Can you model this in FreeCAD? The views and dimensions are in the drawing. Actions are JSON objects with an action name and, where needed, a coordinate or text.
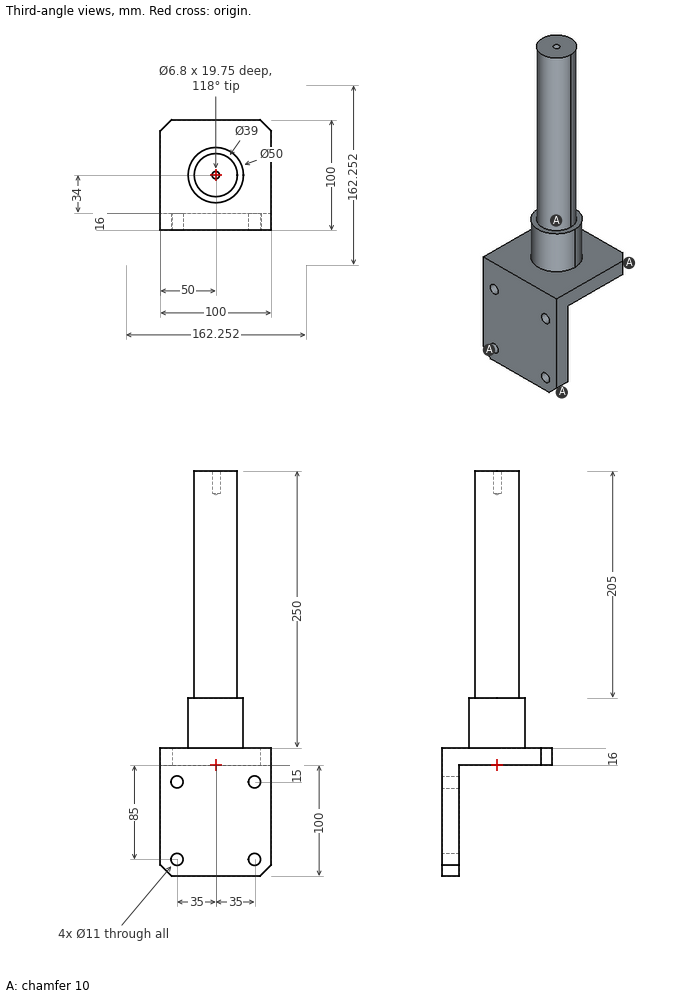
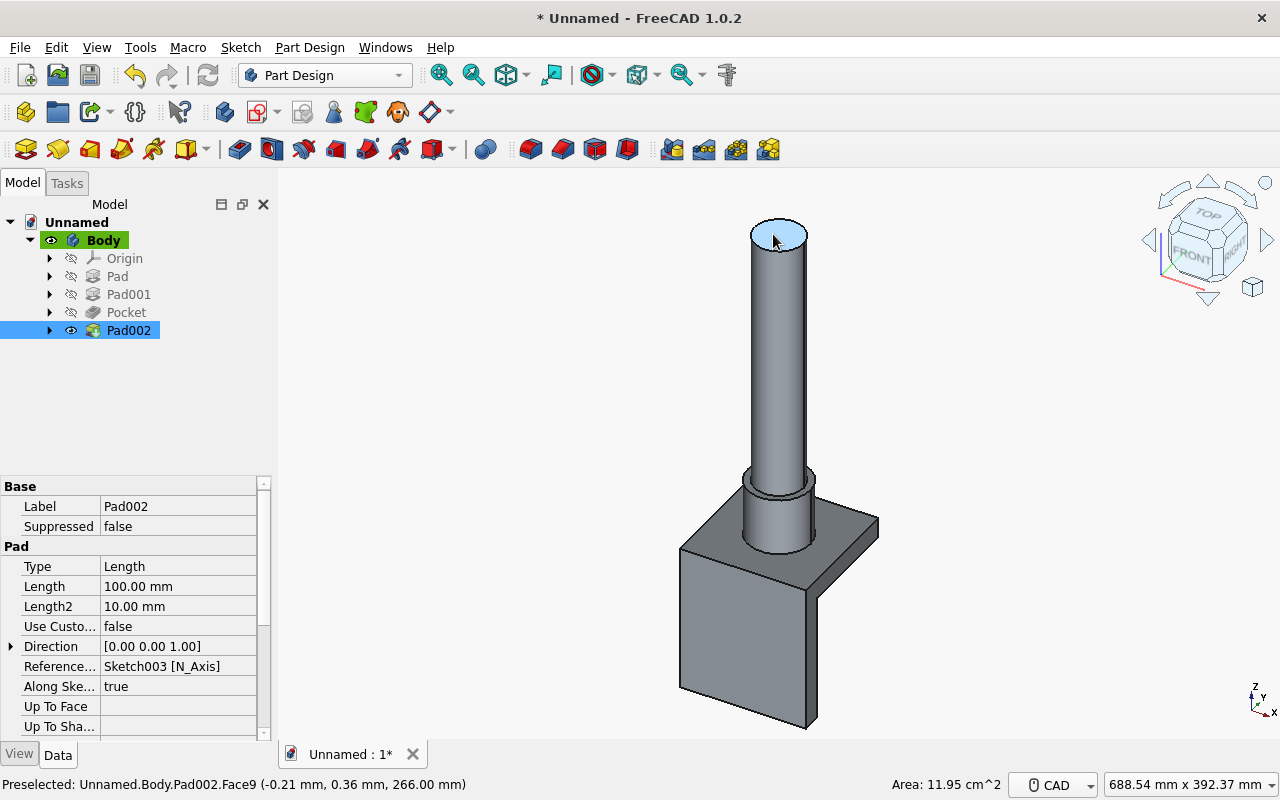
{"action": "left_click", "coordinate": [258, 112]}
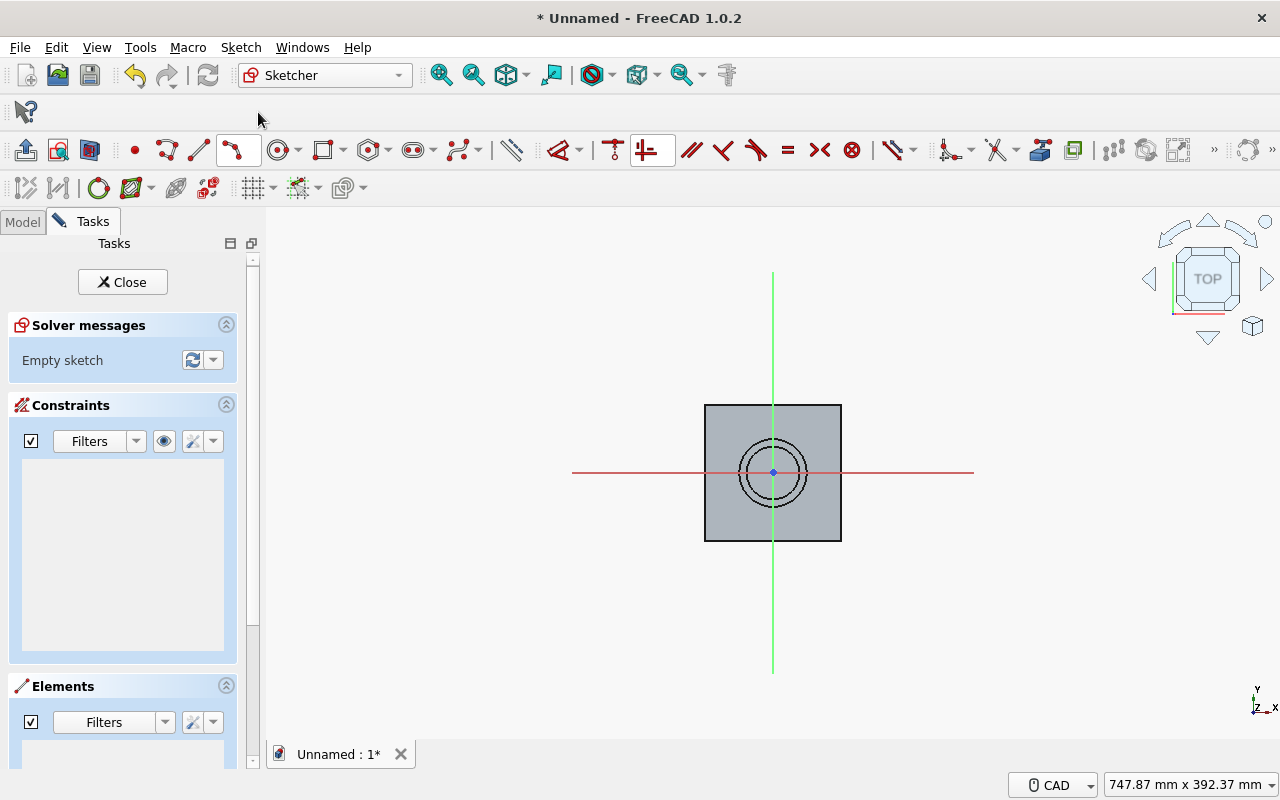
{"action": "scroll", "coordinate": [777, 473], "scroll_direction": "up", "scroll_amount": 15}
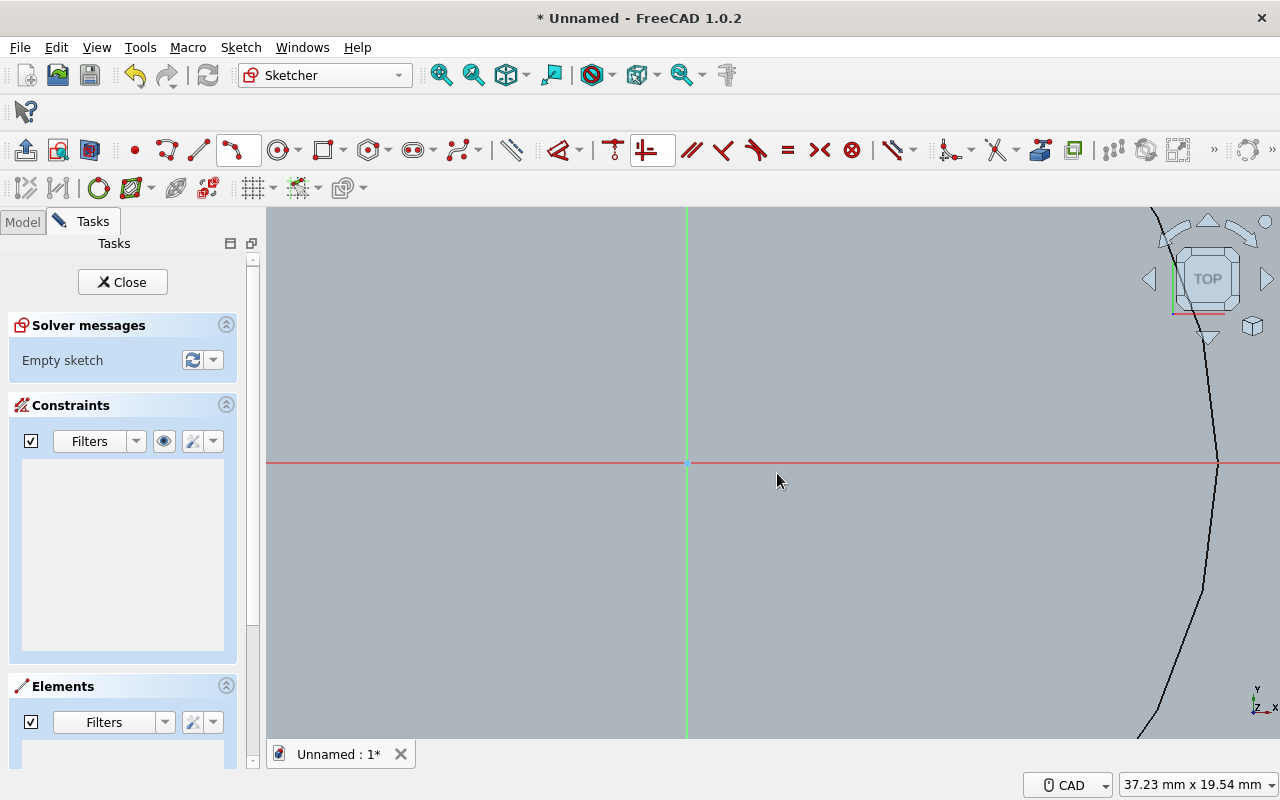
{"action": "scroll", "coordinate": [666, 452], "scroll_direction": "up", "scroll_amount": 3}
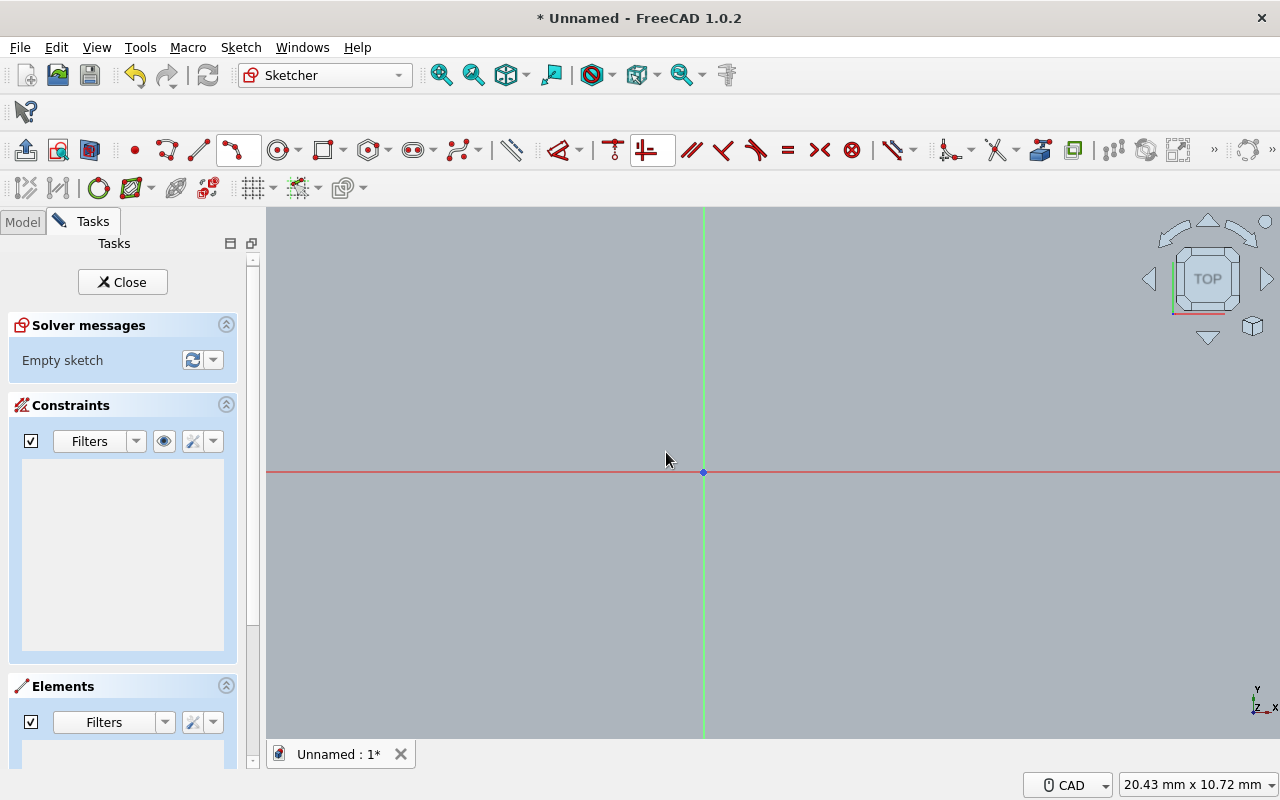
{"action": "left_click", "coordinate": [278, 150]}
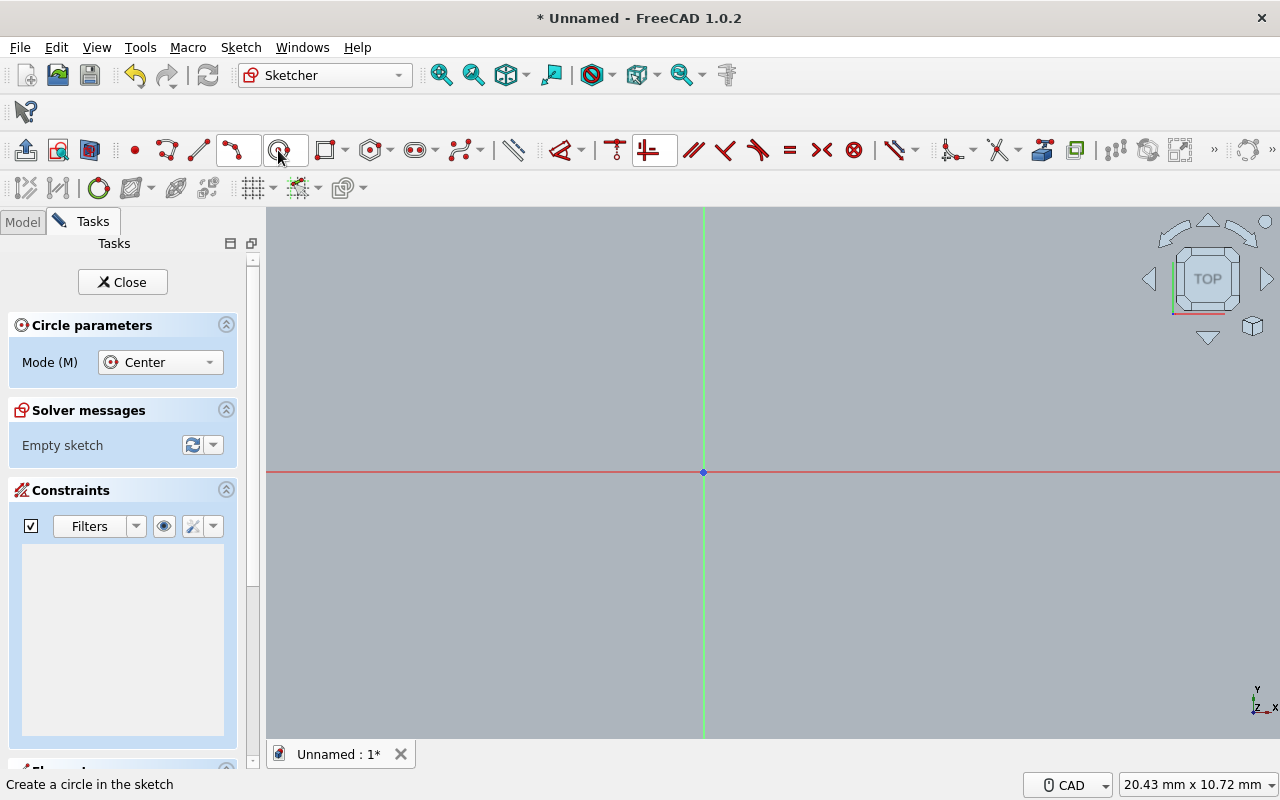
{"action": "left_click", "coordinate": [704, 472]}
{"action": "left_click", "coordinate": [823, 353]}
{"action": "key", "text": "Escape"}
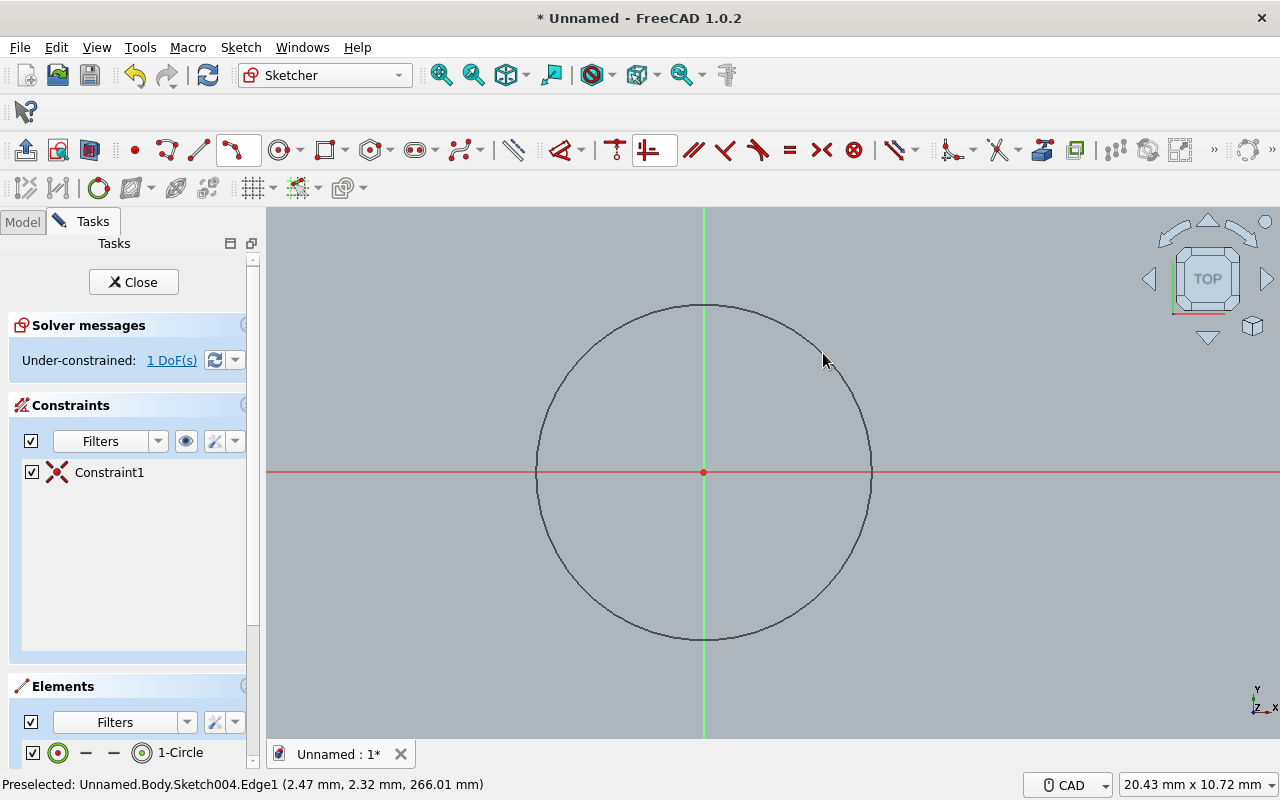
{"action": "key", "text": "d"}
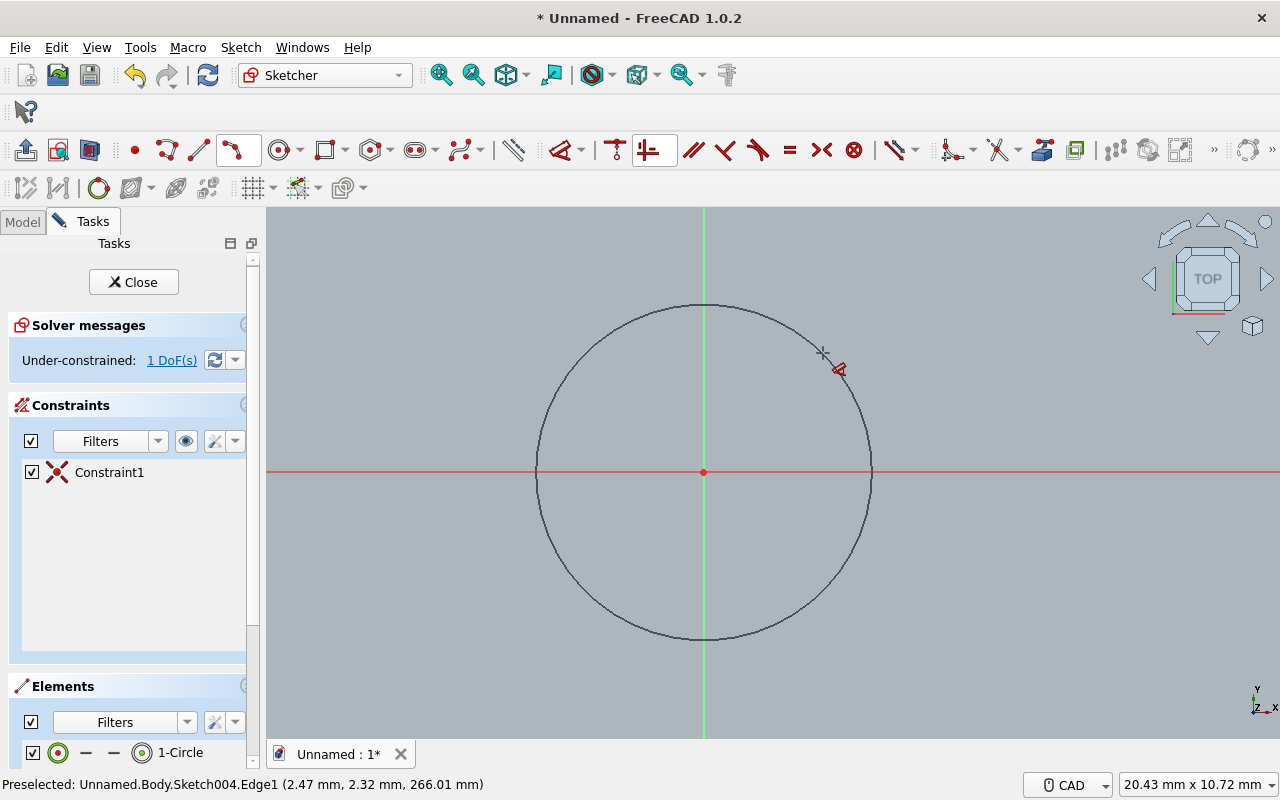
{"action": "left_click", "coordinate": [822, 353]}
{"action": "left_click", "coordinate": [844, 330]}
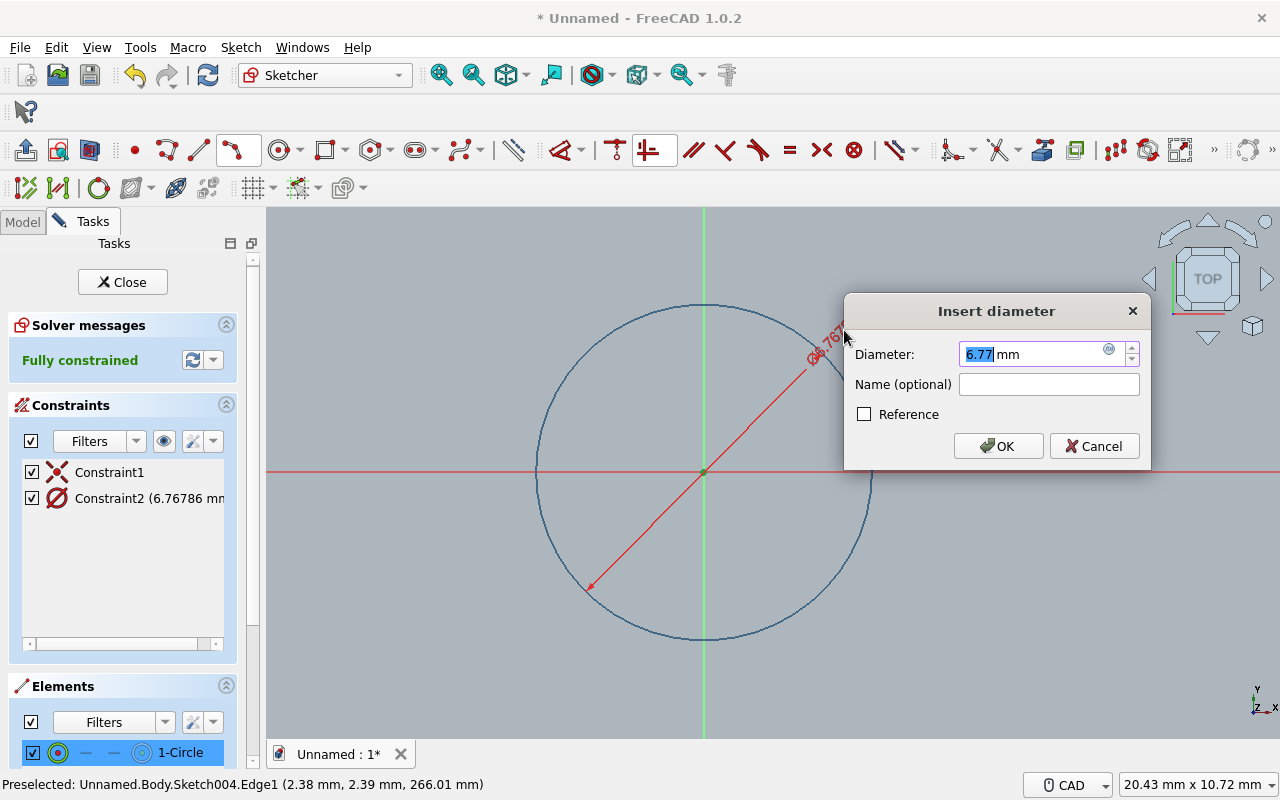
{"action": "type", "text": "6.8"}
{"action": "key", "text": "Return"}
{"action": "key", "text": "Escape"}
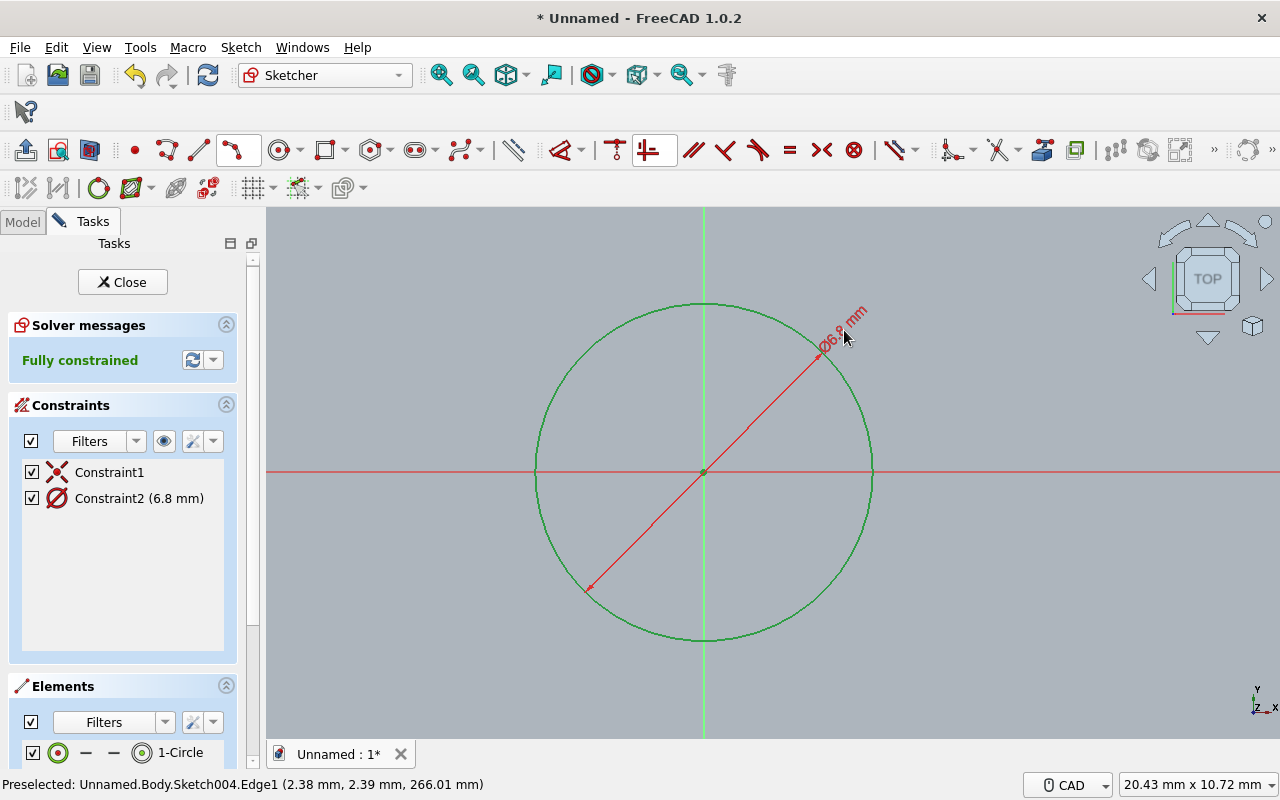
{"action": "left_click", "coordinate": [123, 282]}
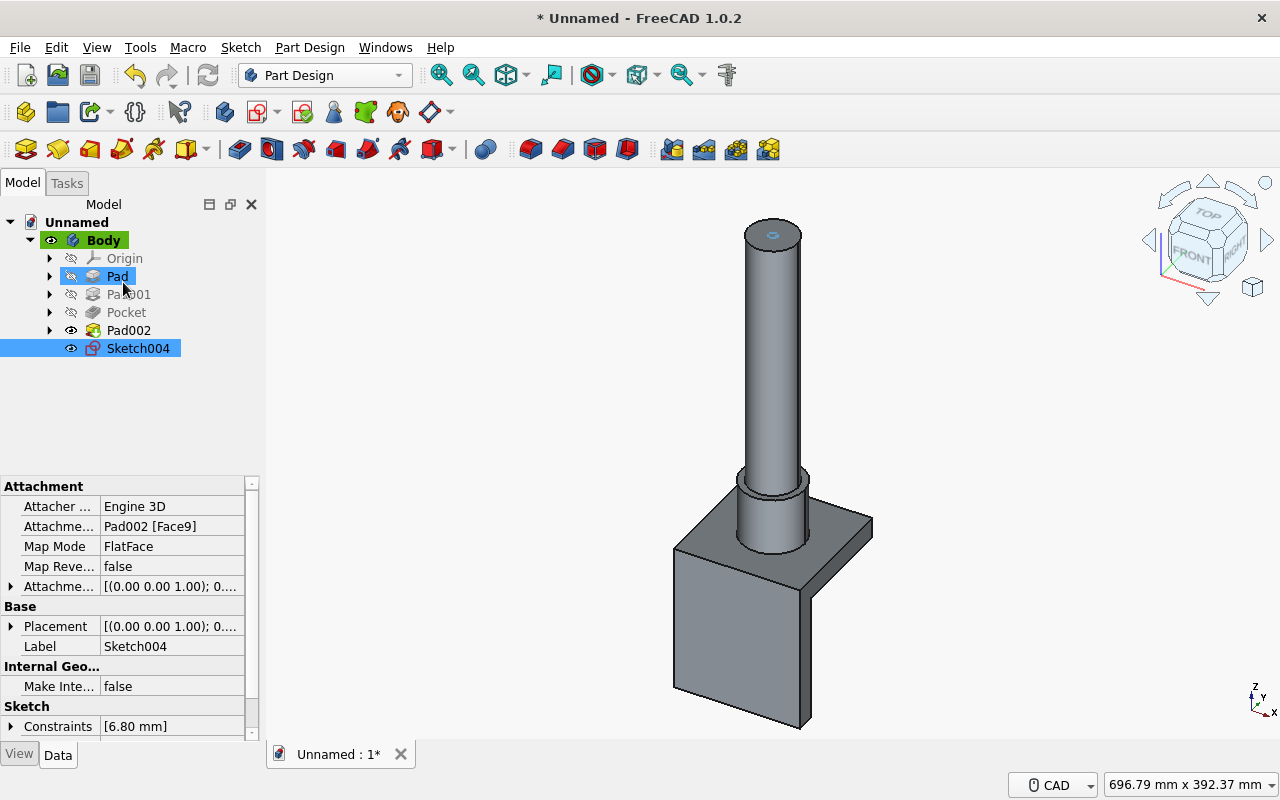
{"action": "left_click", "coordinate": [272, 150]}